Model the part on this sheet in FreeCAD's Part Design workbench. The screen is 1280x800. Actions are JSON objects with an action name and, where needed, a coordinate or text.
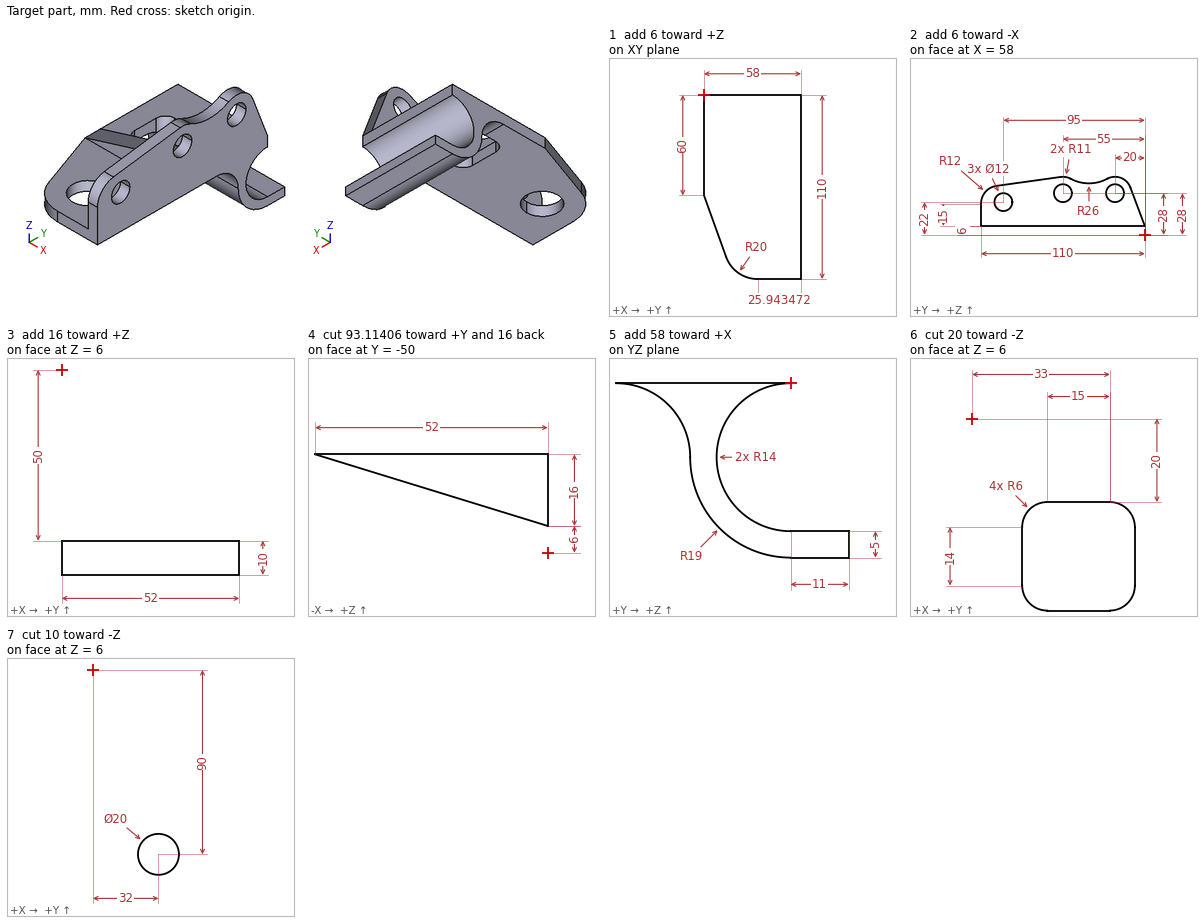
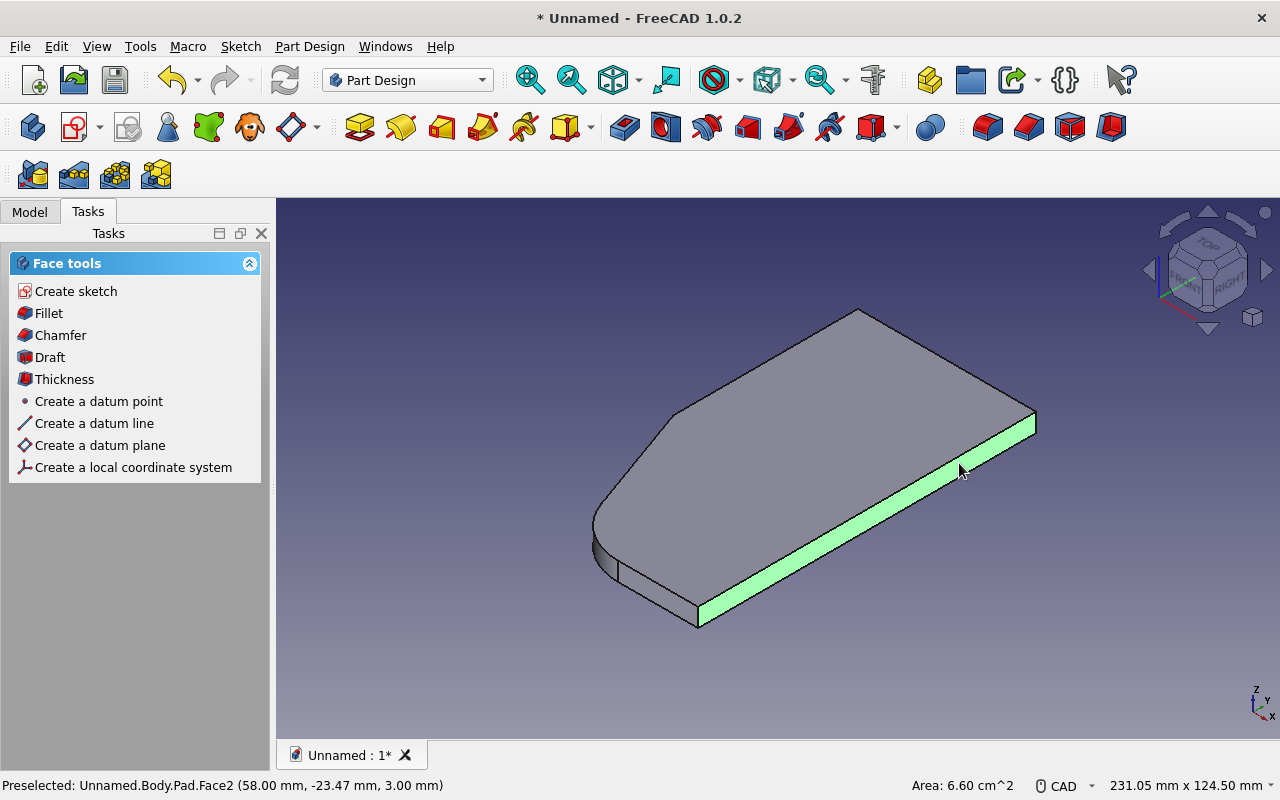
{"action": "left_click", "coordinate": [74, 128]}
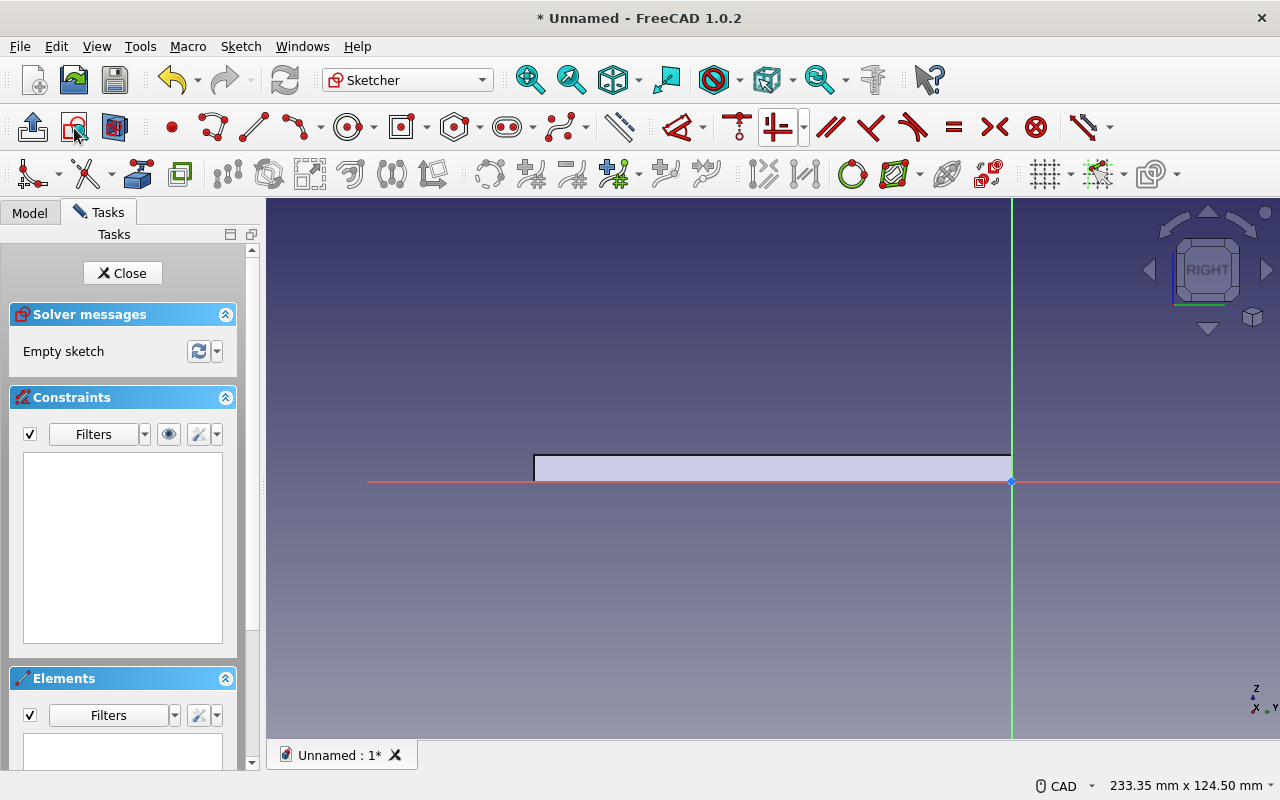
{"action": "left_click", "coordinate": [213, 128]}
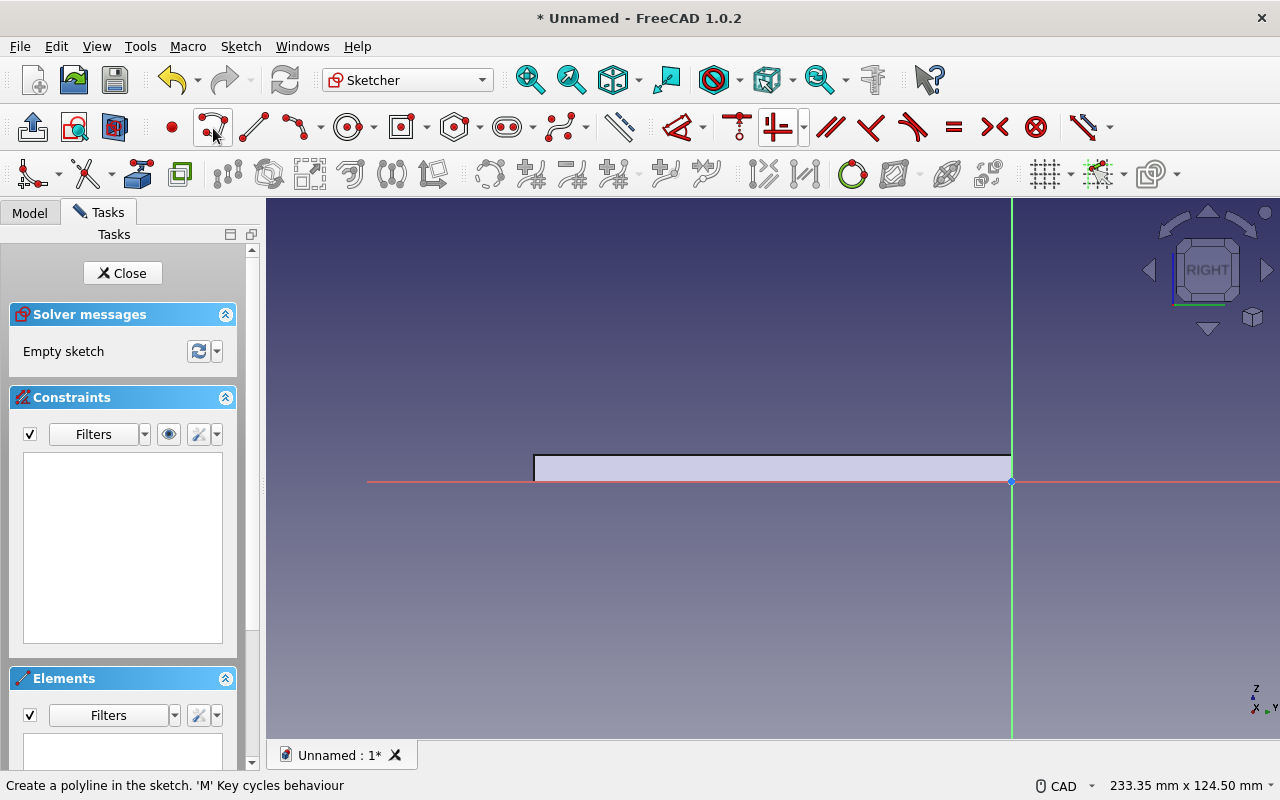
{"action": "left_click", "coordinate": [534, 390]}
{"action": "left_click", "coordinate": [534, 455]}
{"action": "left_click", "coordinate": [1012, 455]}
{"action": "left_click", "coordinate": [970, 343]}
{"action": "right_click", "coordinate": [970, 343]}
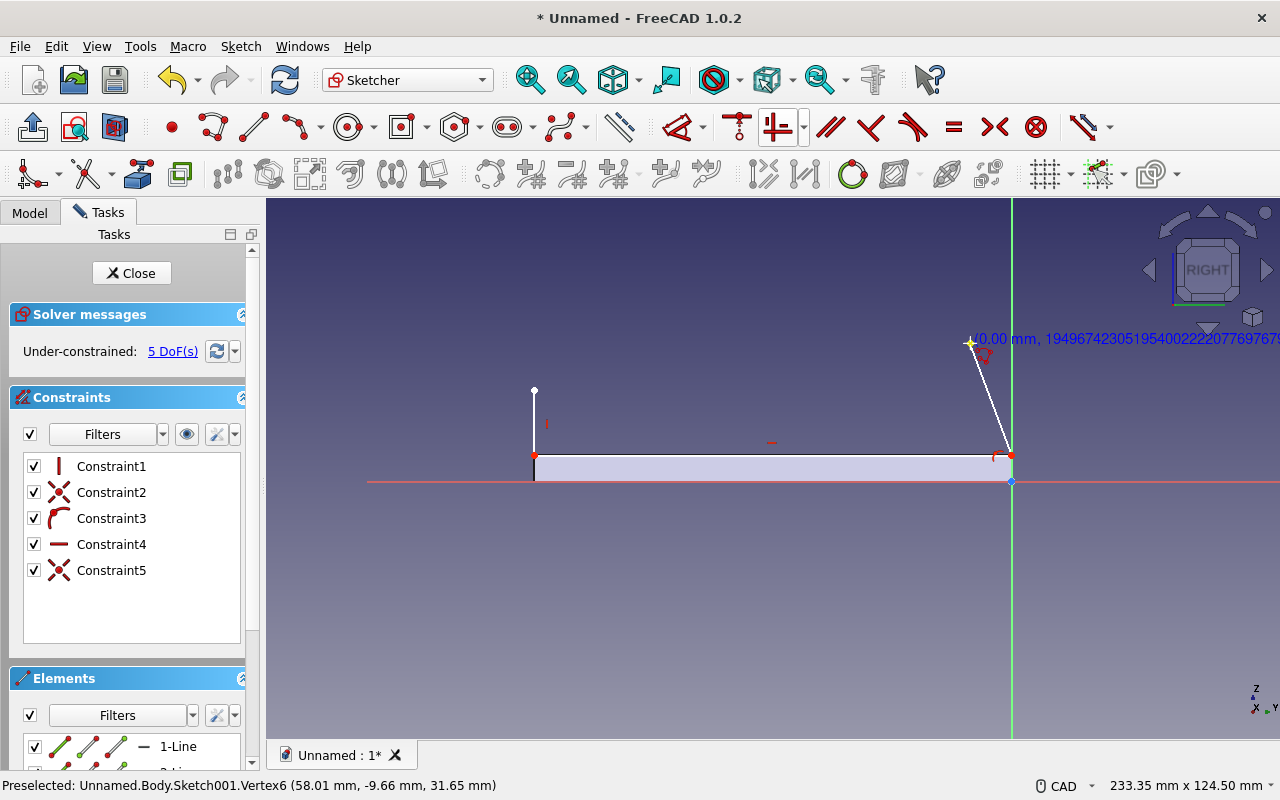
{"action": "left_click", "coordinate": [254, 128]}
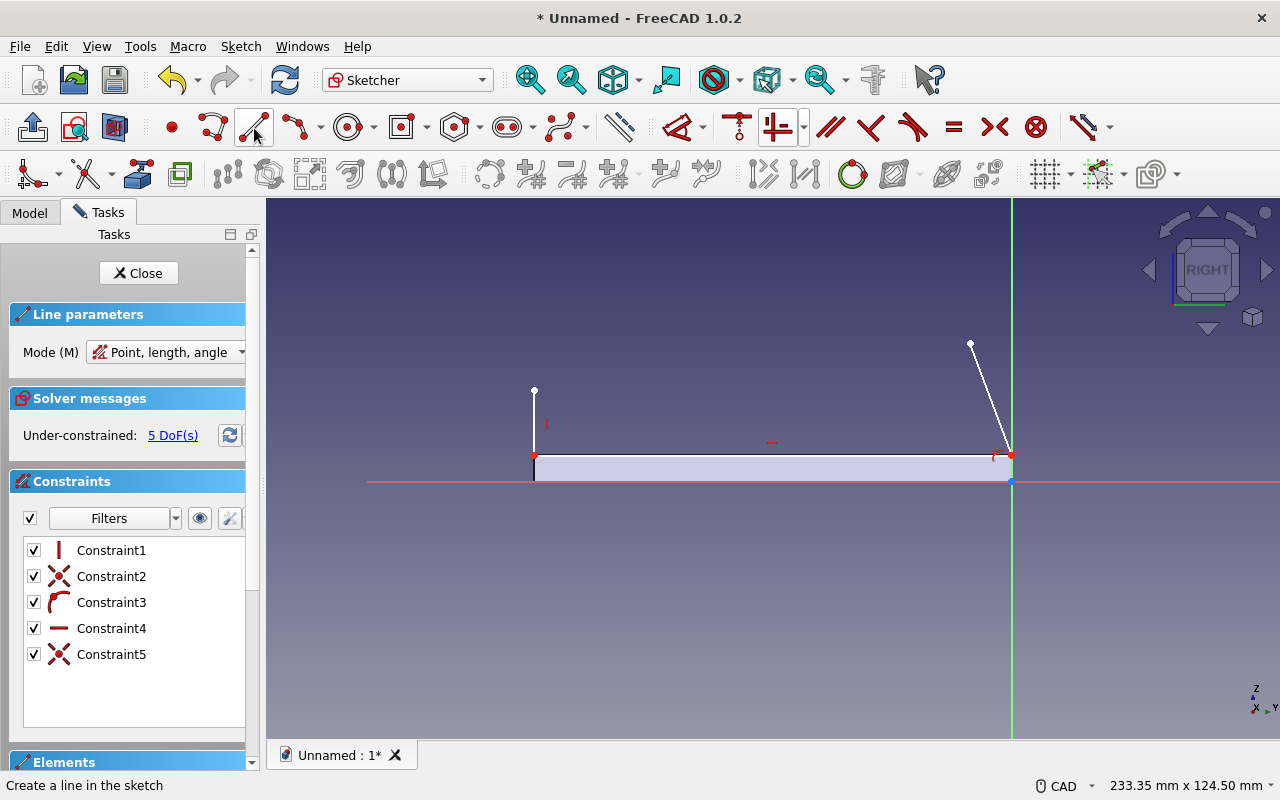
{"action": "left_click", "coordinate": [766, 313]}
{"action": "left_click", "coordinate": [579, 339]}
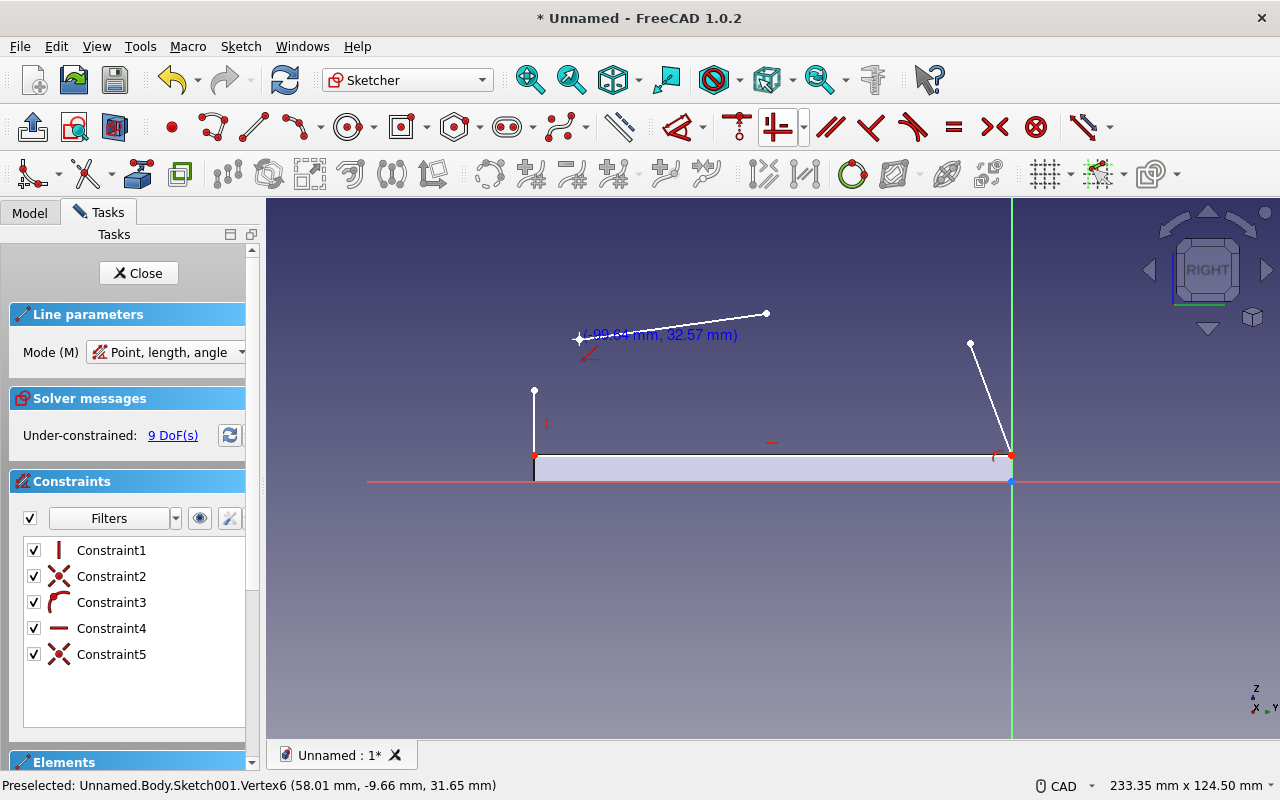
{"action": "left_click", "coordinate": [294, 128]}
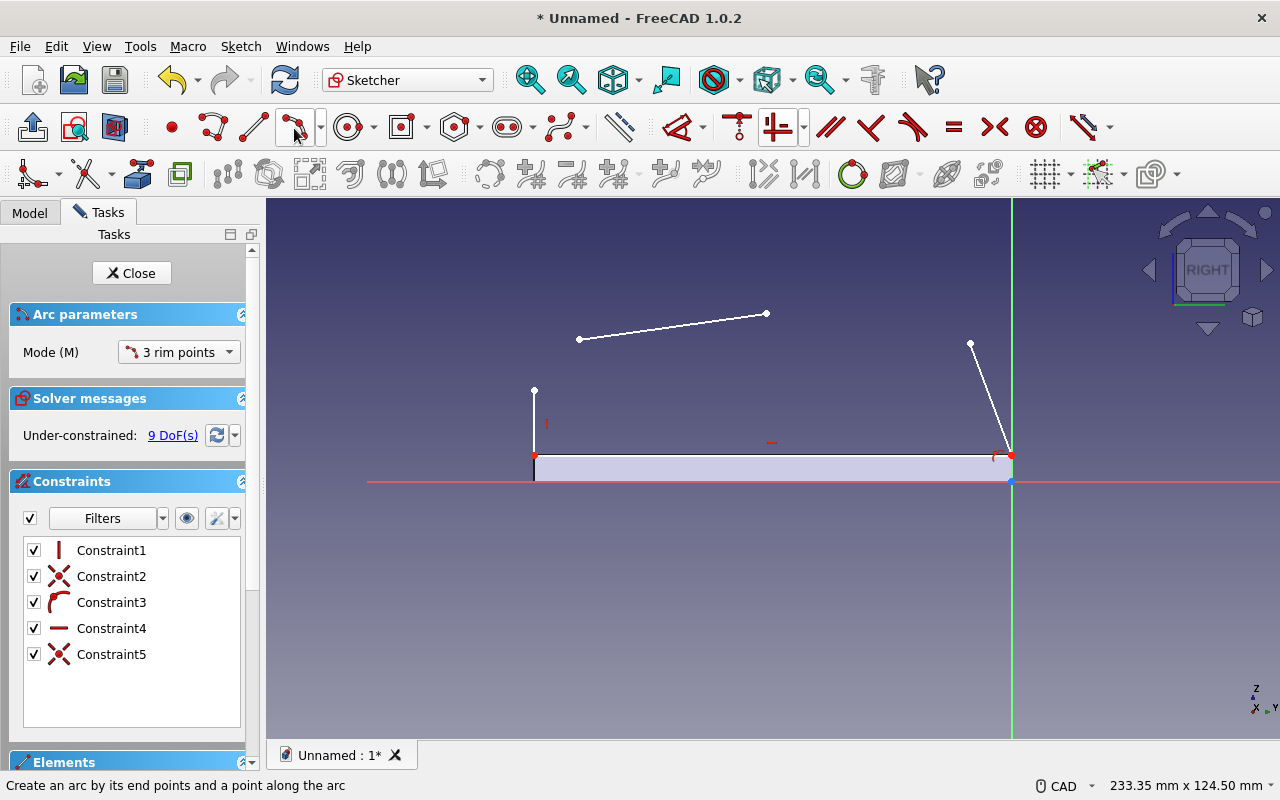
{"action": "left_click", "coordinate": [970, 344]}
{"action": "left_click", "coordinate": [902, 318]}
{"action": "left_click", "coordinate": [942, 315]}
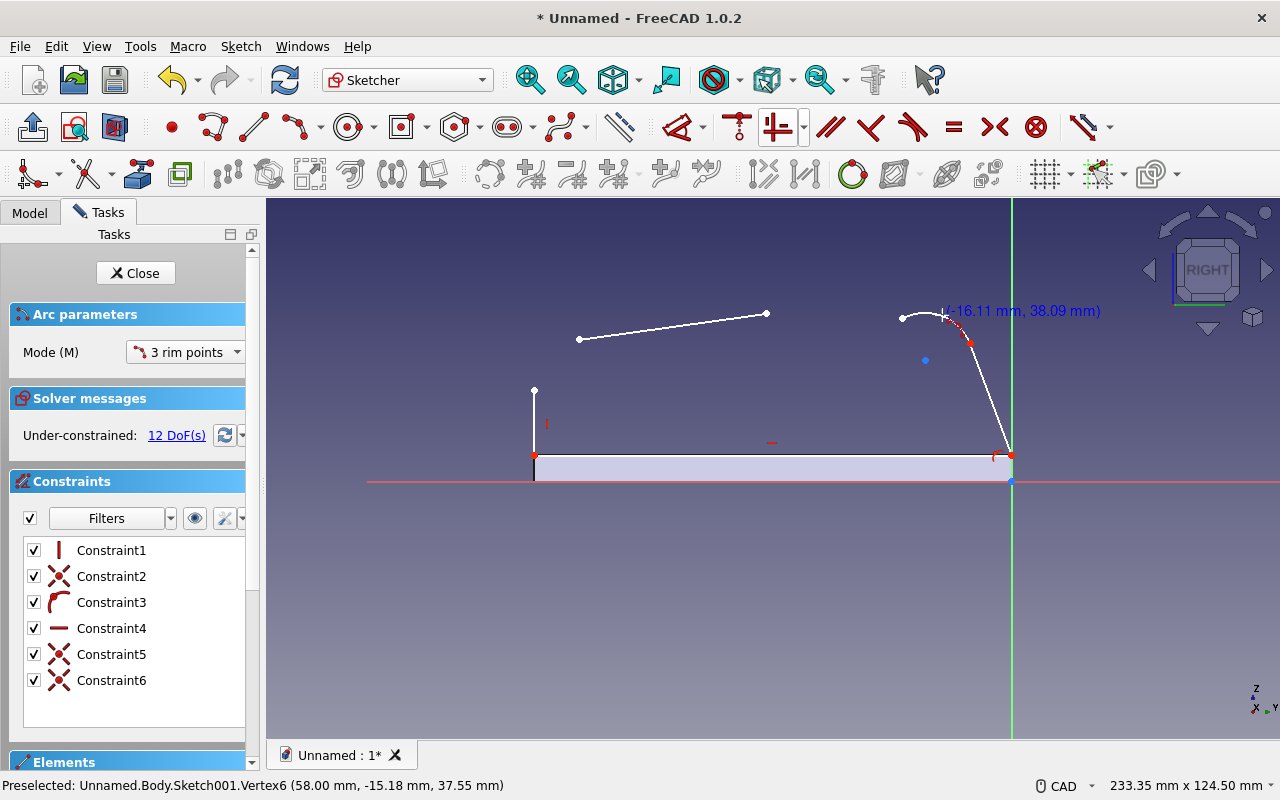
{"action": "left_click", "coordinate": [902, 319]}
{"action": "left_click", "coordinate": [796, 318]}
{"action": "left_click", "coordinate": [849, 331]}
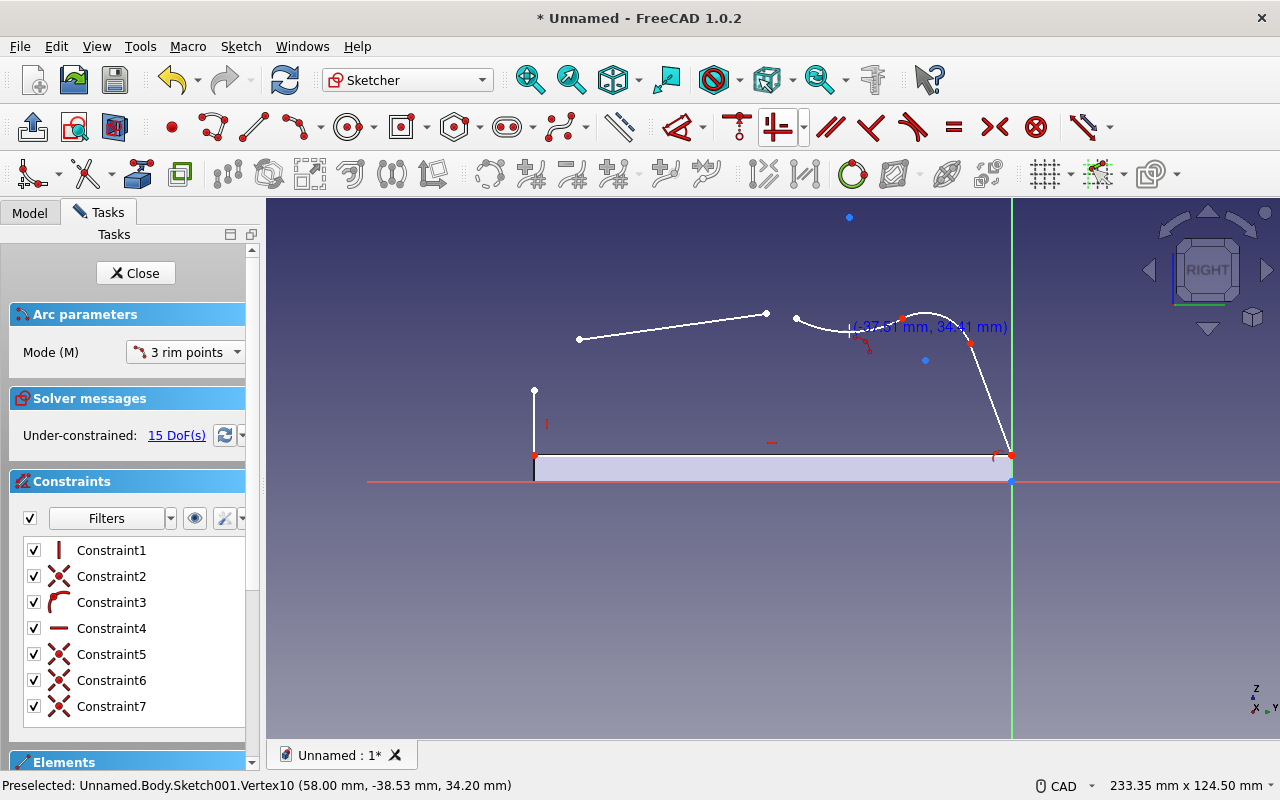
{"action": "left_click", "coordinate": [796, 319]}
{"action": "left_click", "coordinate": [766, 314]}